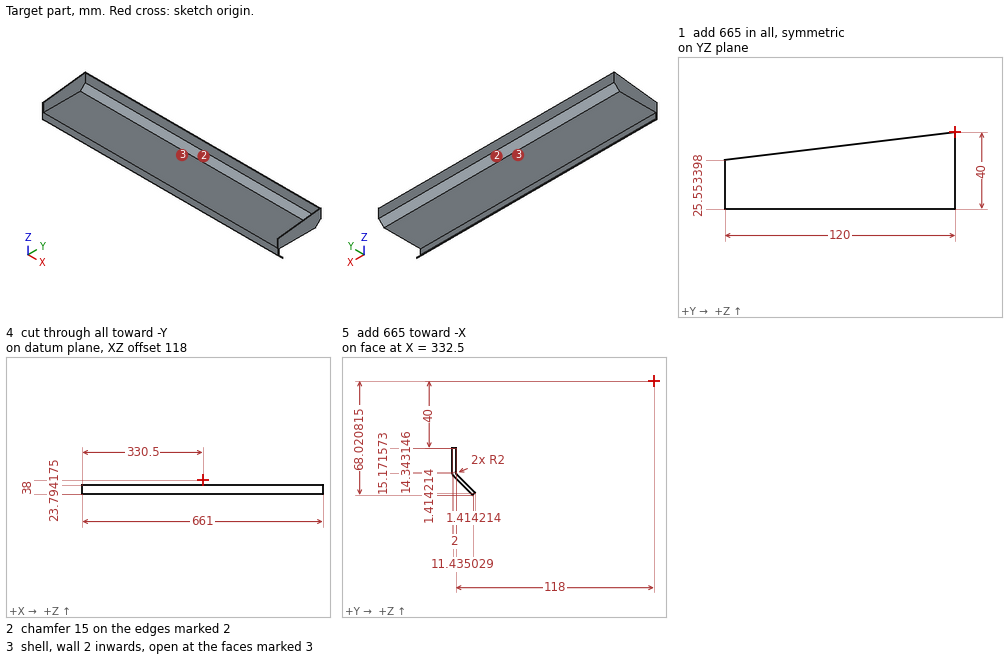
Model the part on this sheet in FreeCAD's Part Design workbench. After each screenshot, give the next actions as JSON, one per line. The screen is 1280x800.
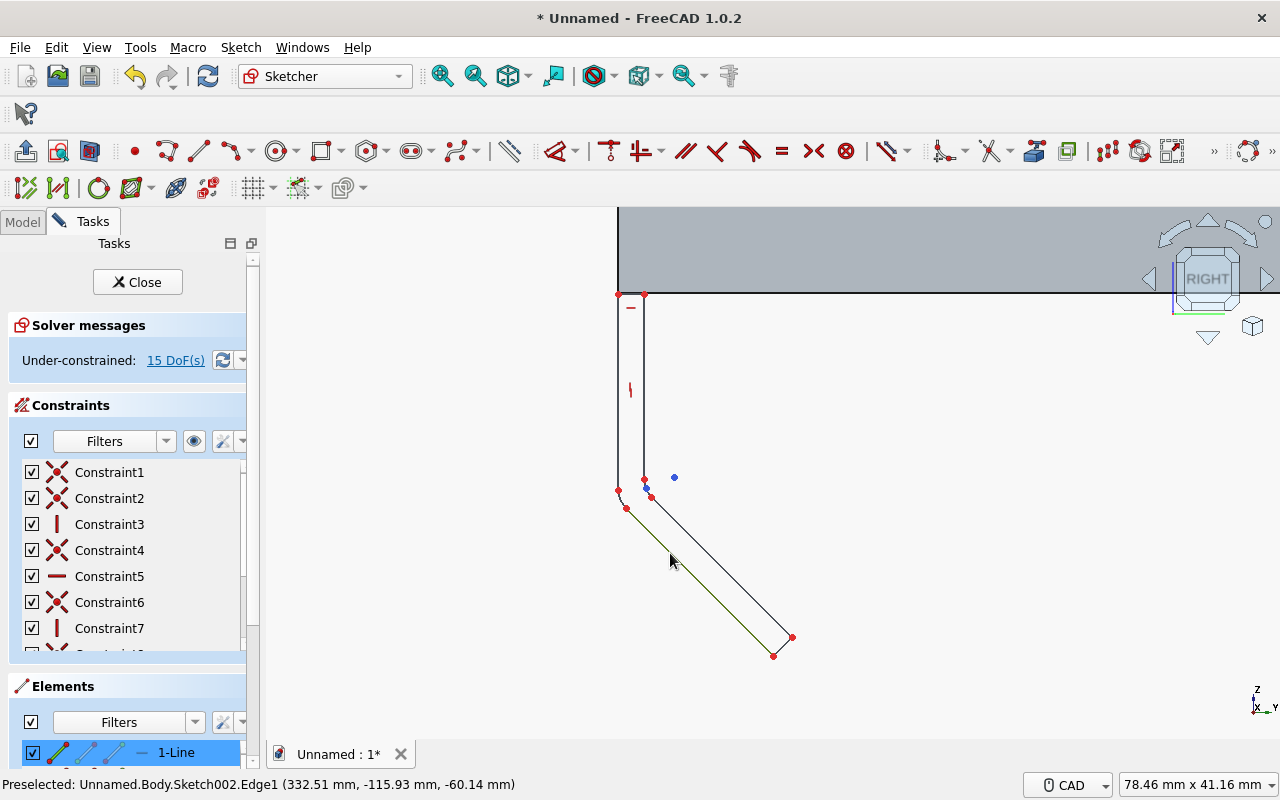
{"action": "scroll", "coordinate": [621, 500], "scroll_direction": "up", "scroll_amount": 2}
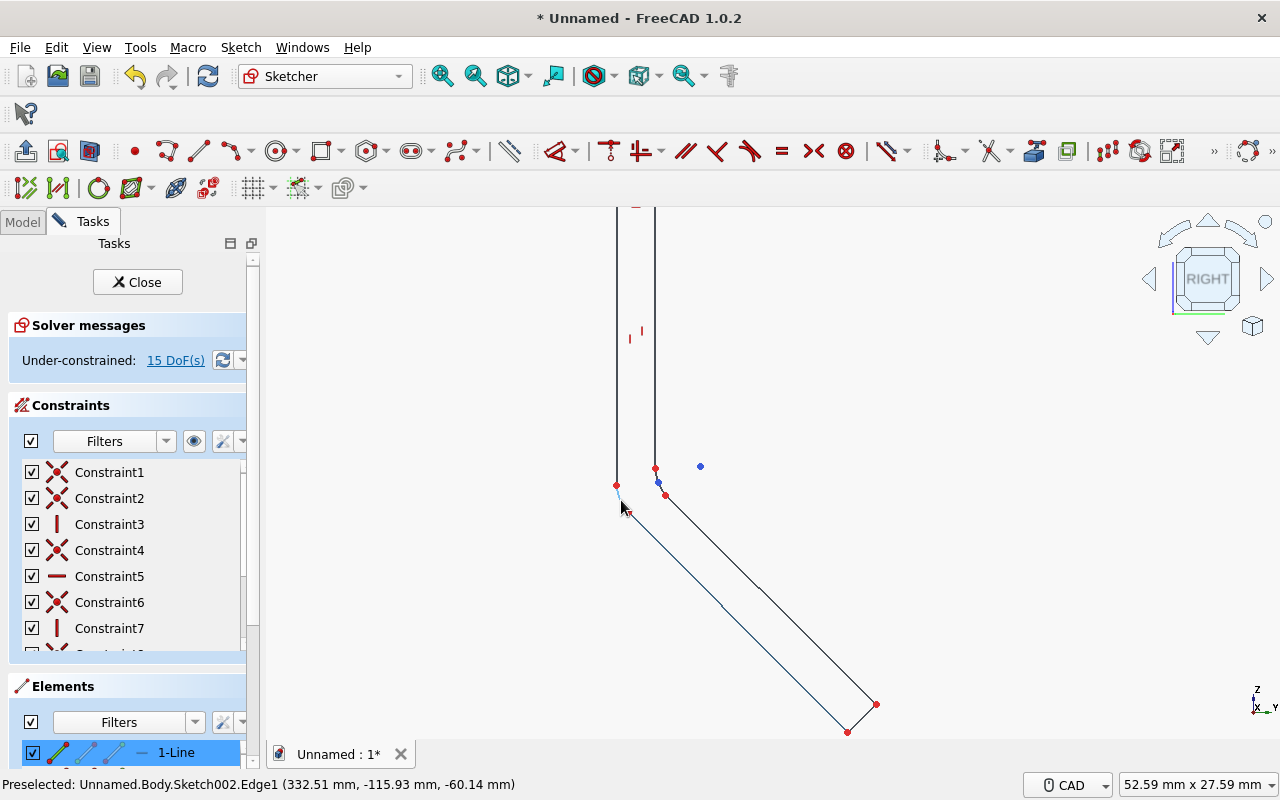
{"action": "left_click", "coordinate": [620, 500]}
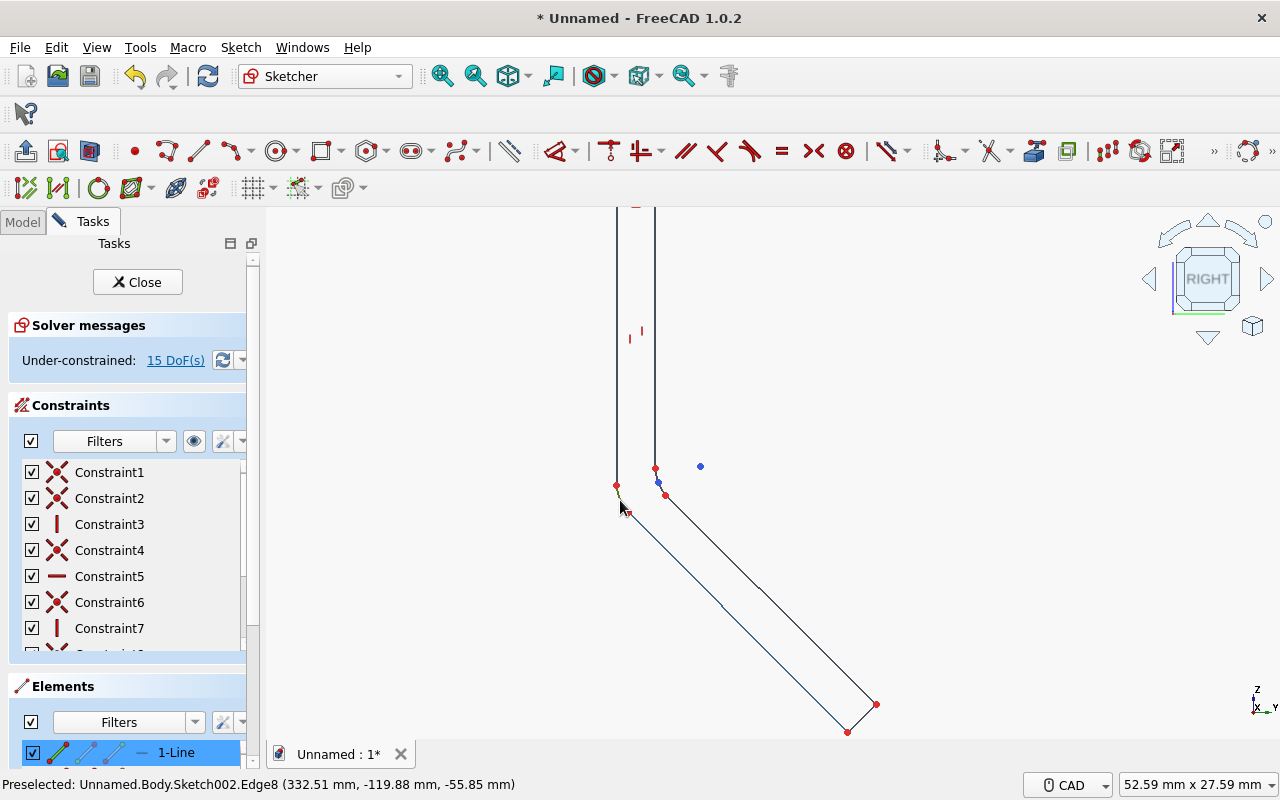
{"action": "left_click", "coordinate": [750, 152]}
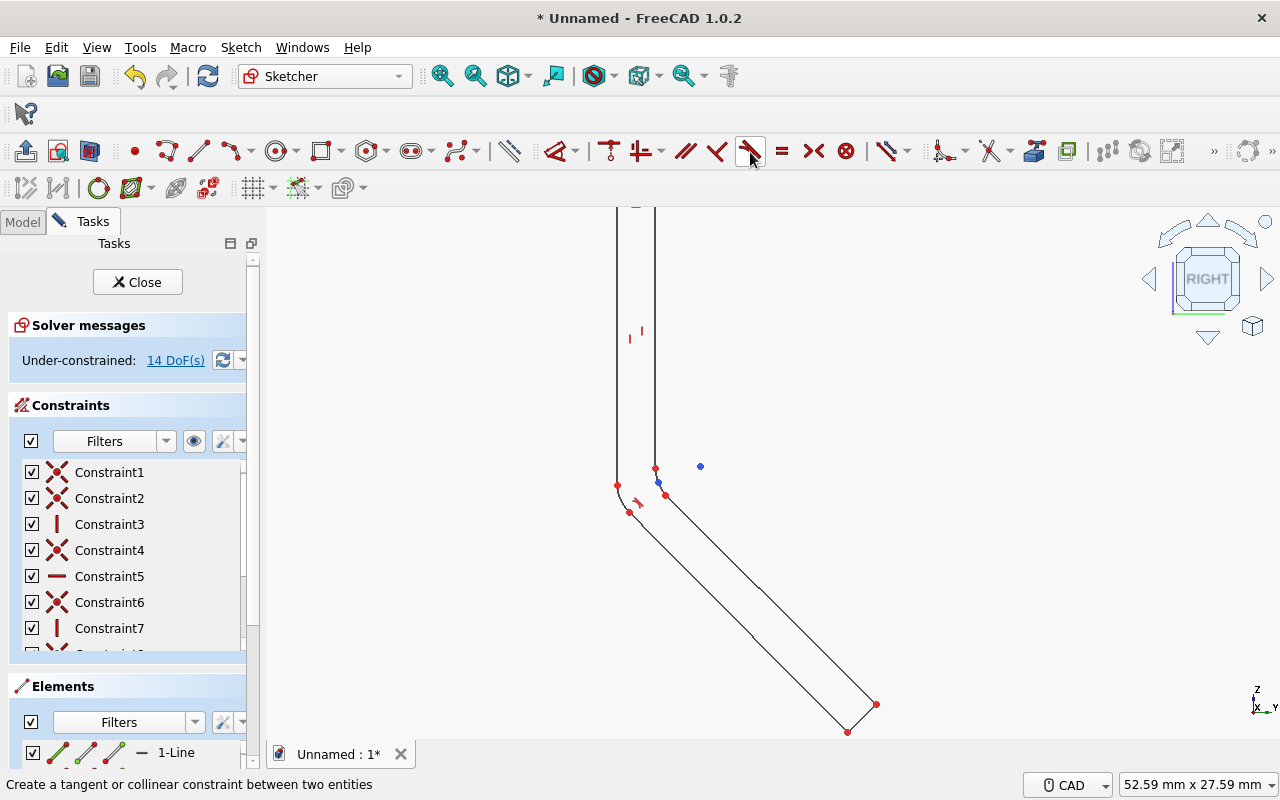
{"action": "left_click", "coordinate": [813, 642]}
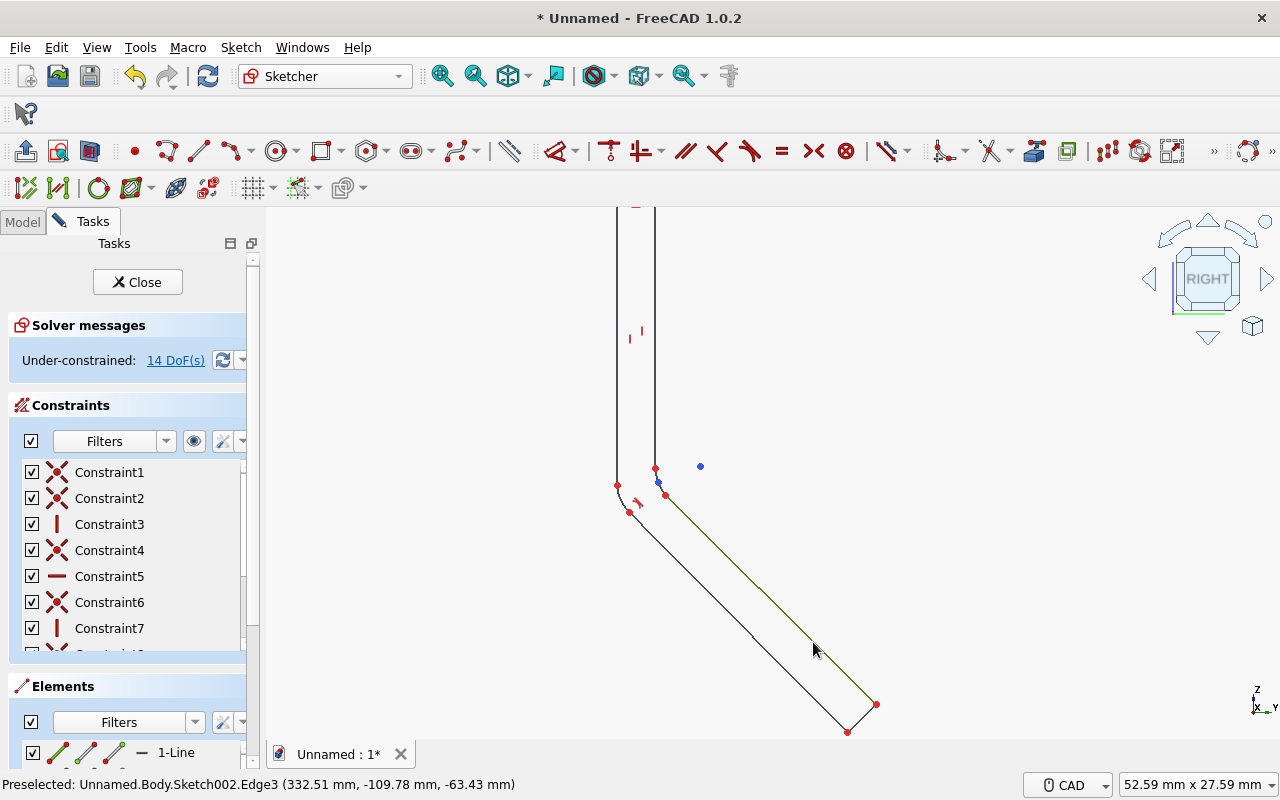
{"action": "left_click", "coordinate": [661, 488]}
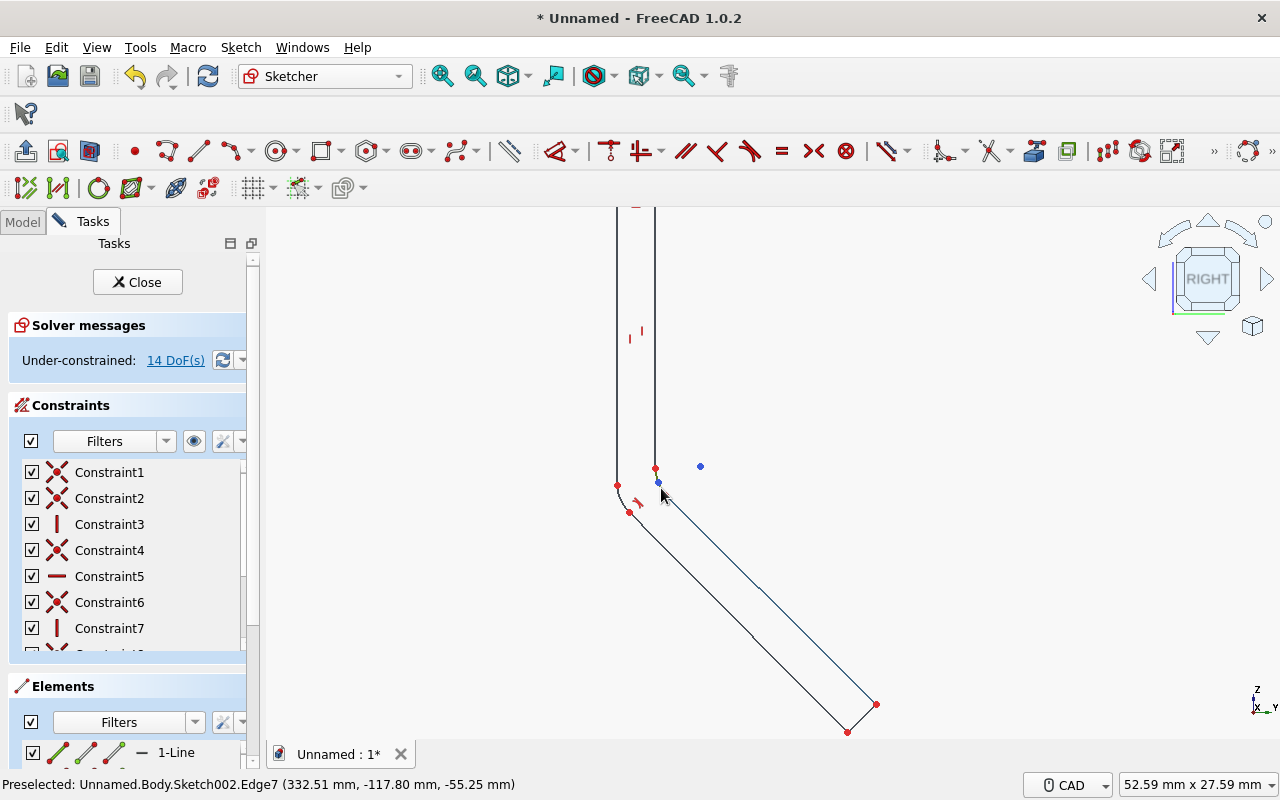
{"action": "key", "text": "t"}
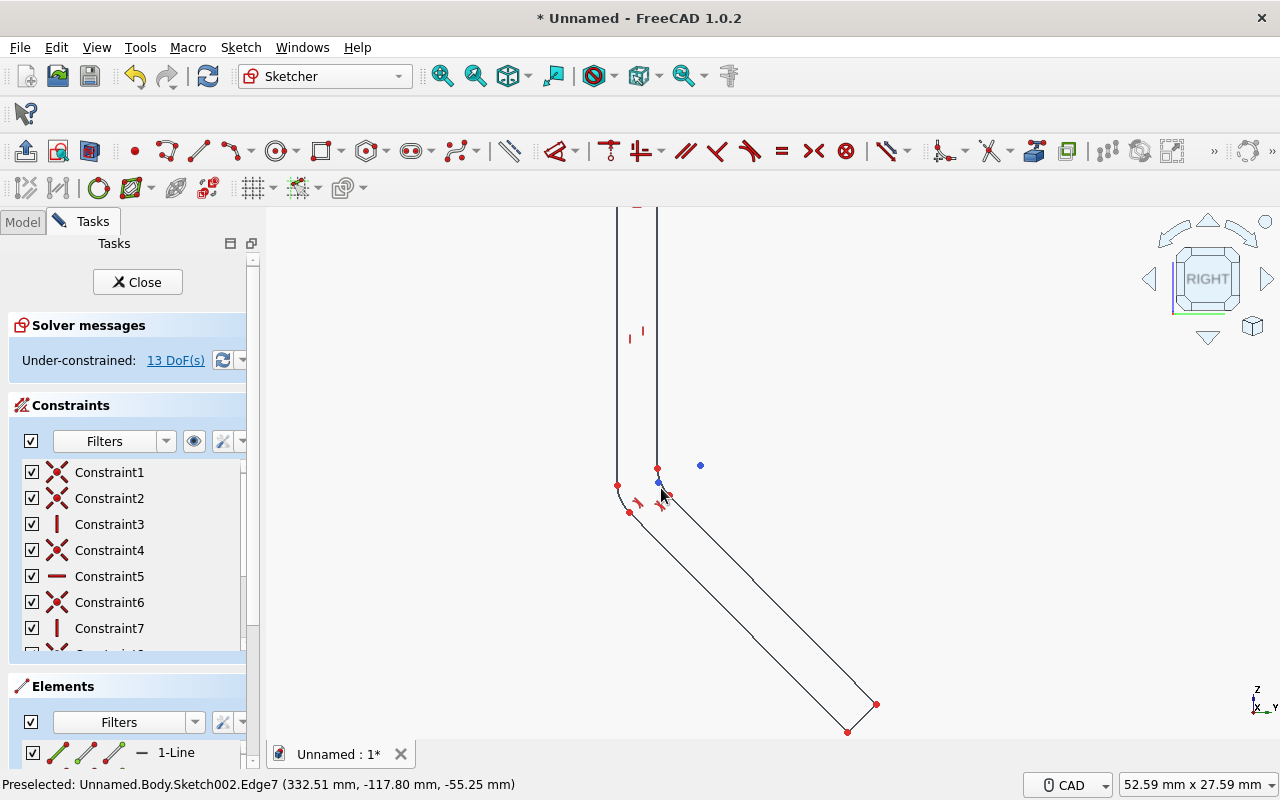
{"action": "left_click", "coordinate": [657, 386]}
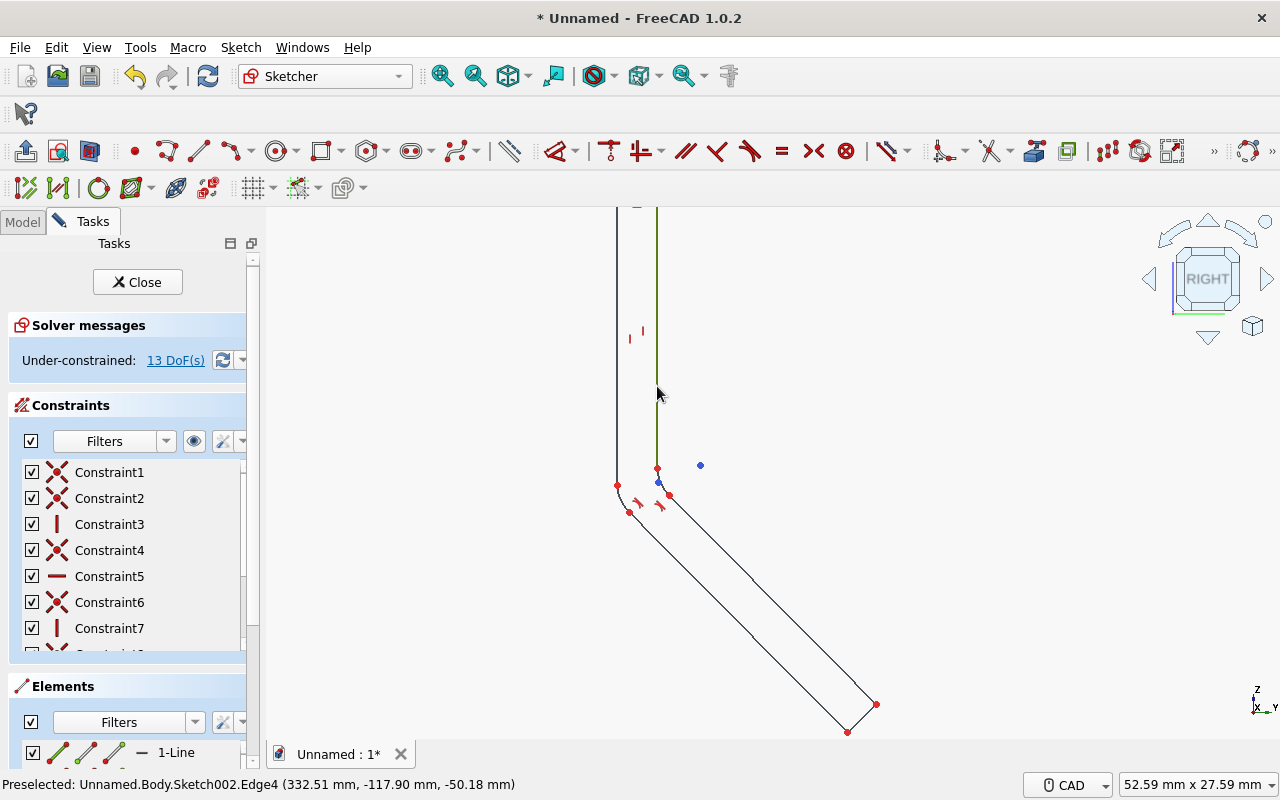
{"action": "scroll", "coordinate": [659, 478], "scroll_direction": "up", "scroll_amount": 3}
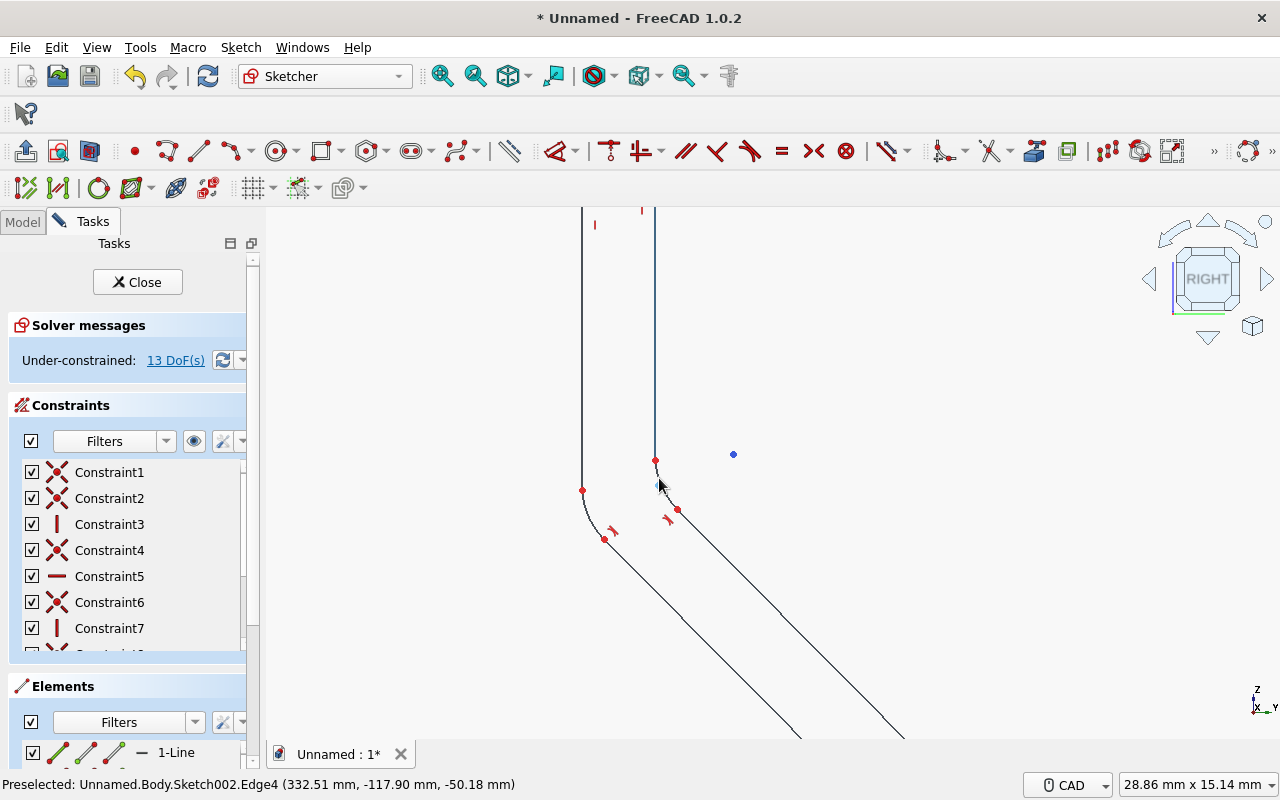
{"action": "left_click", "coordinate": [658, 477]}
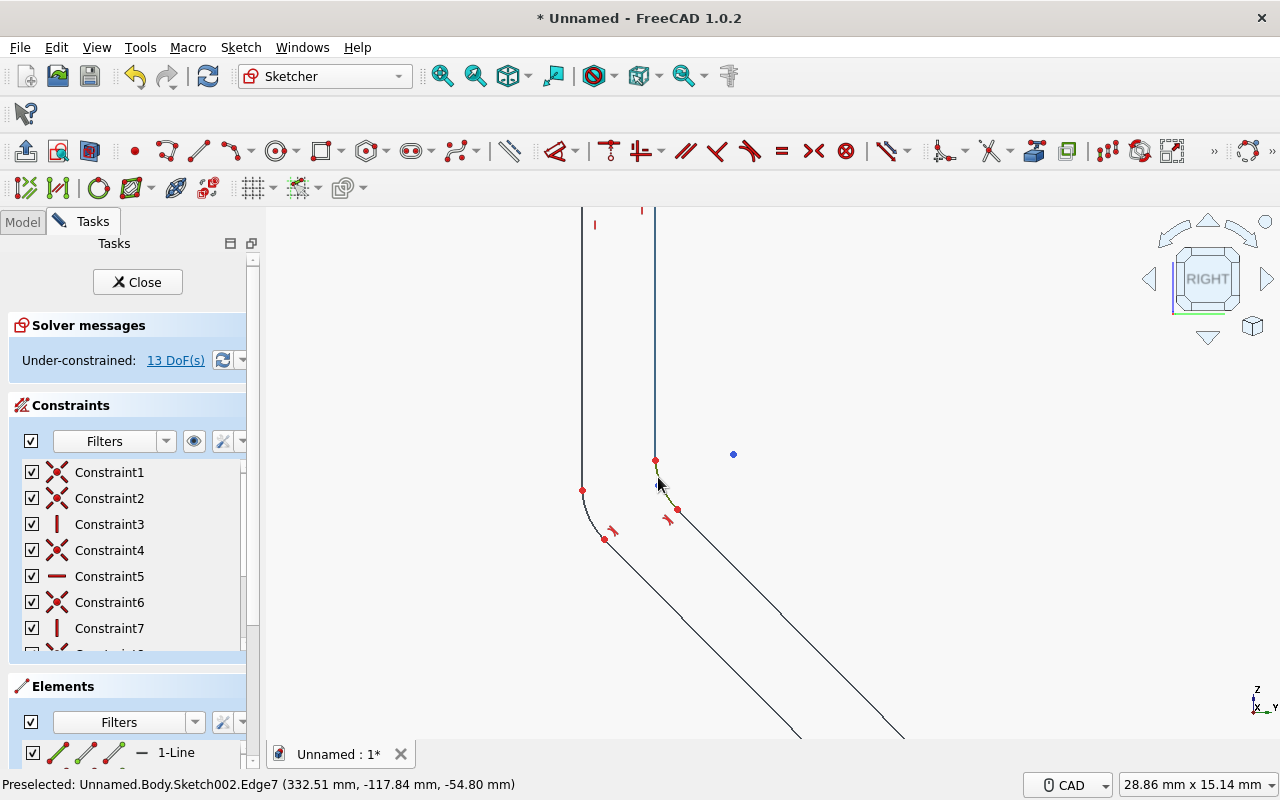
{"action": "key", "text": "t"}